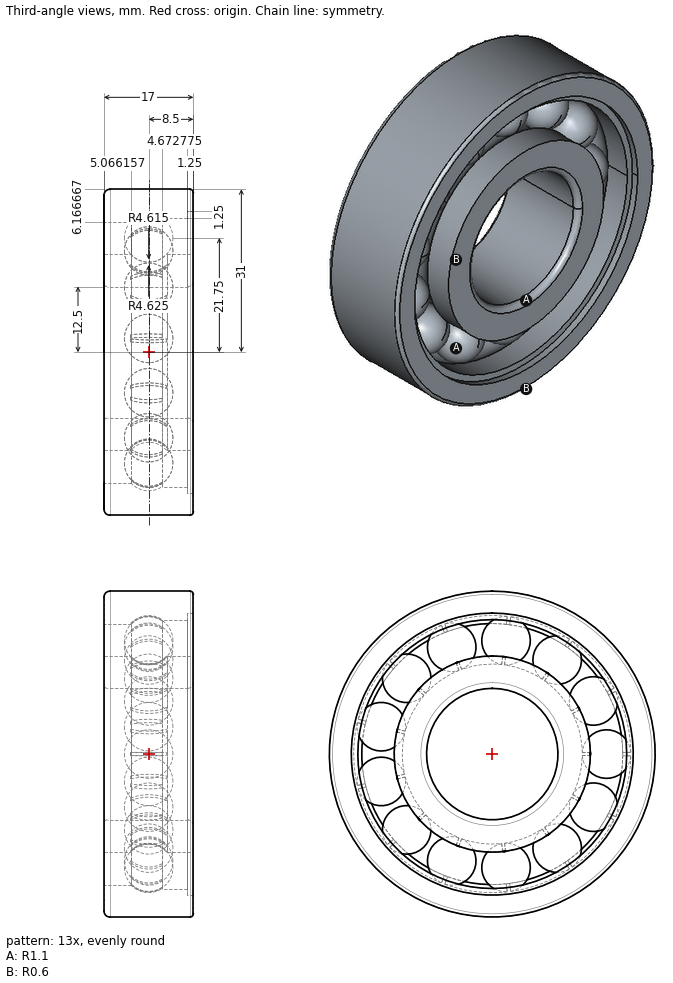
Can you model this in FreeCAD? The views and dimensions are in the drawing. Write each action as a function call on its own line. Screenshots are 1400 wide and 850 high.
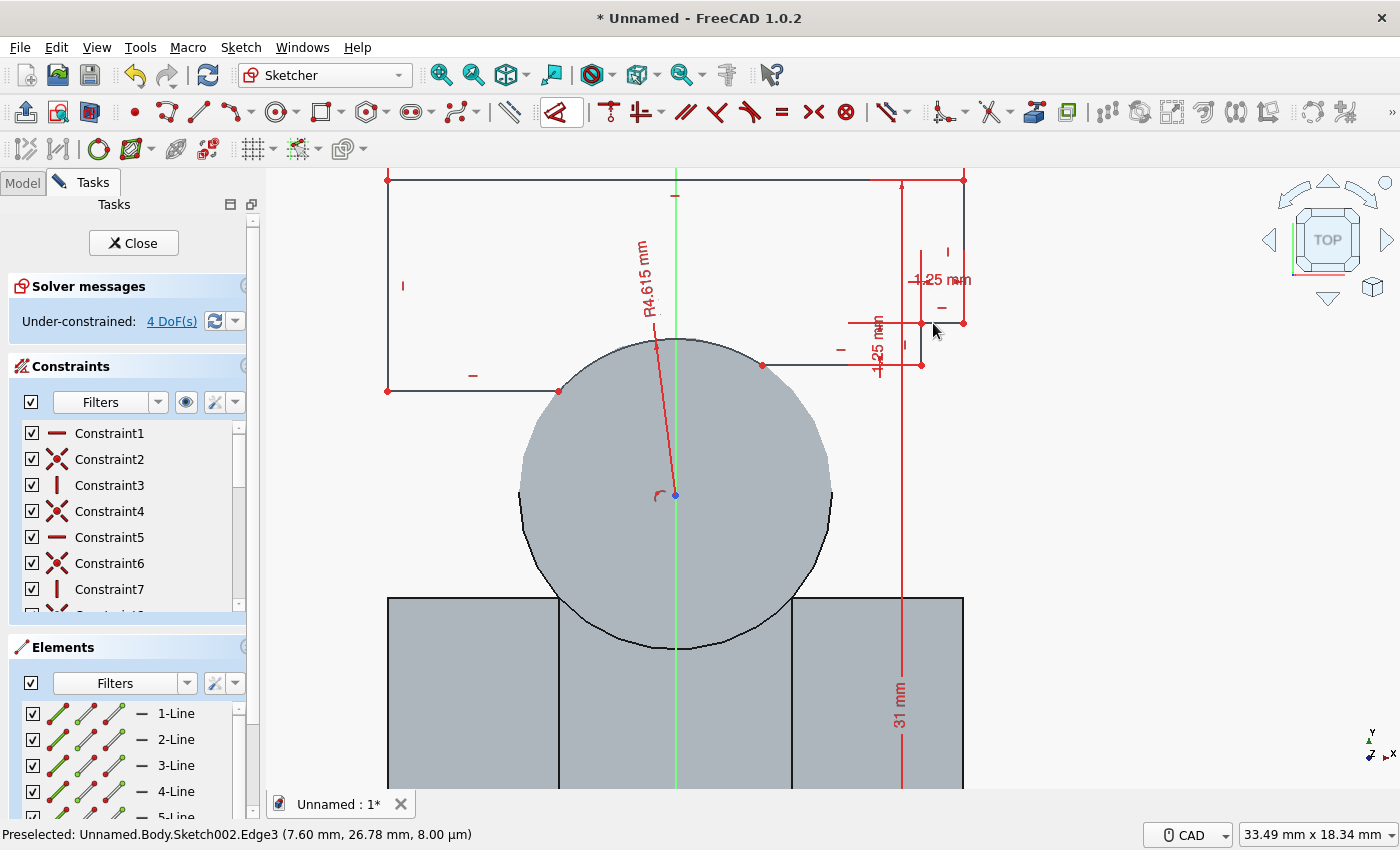
click(964, 323)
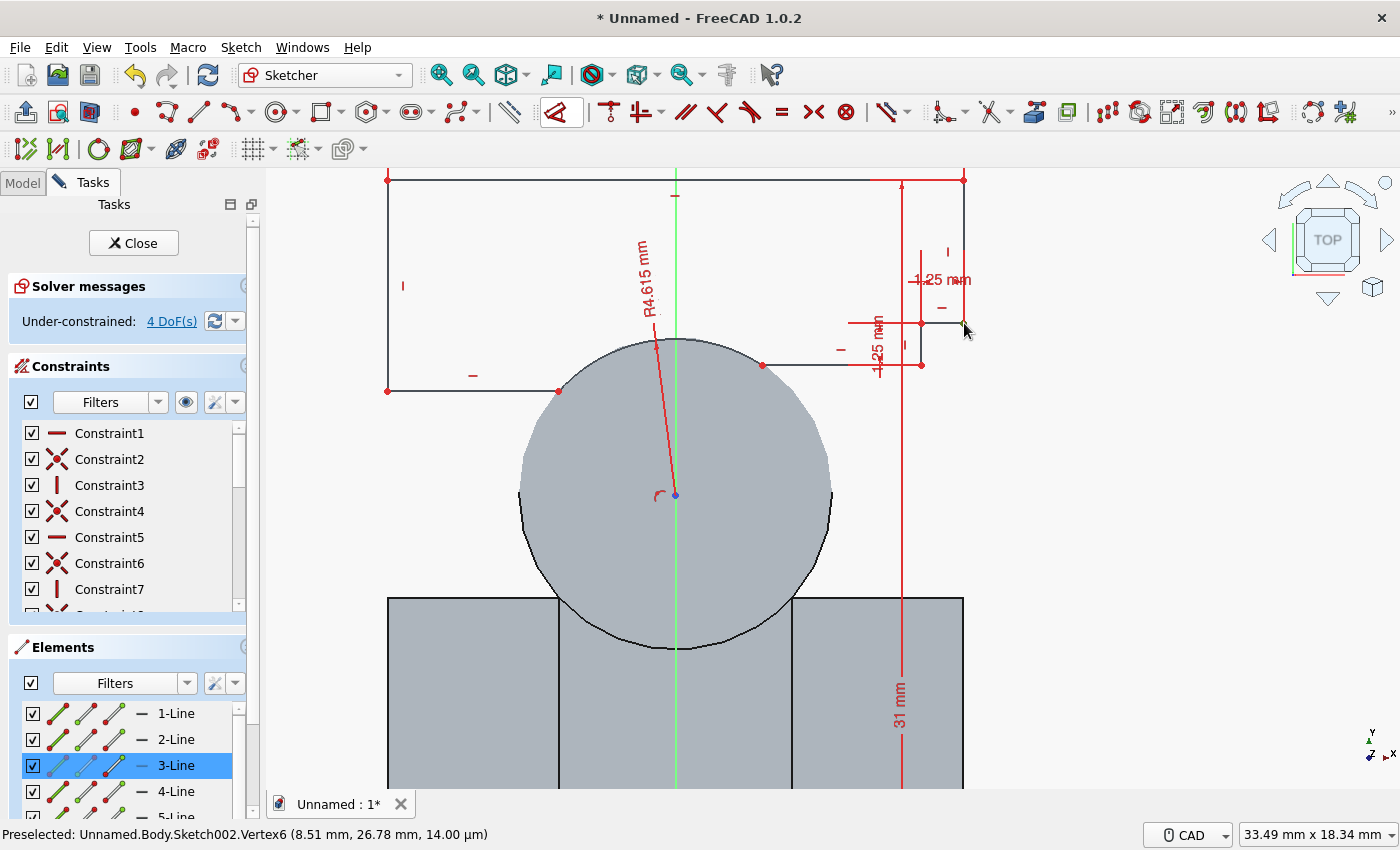
key(l)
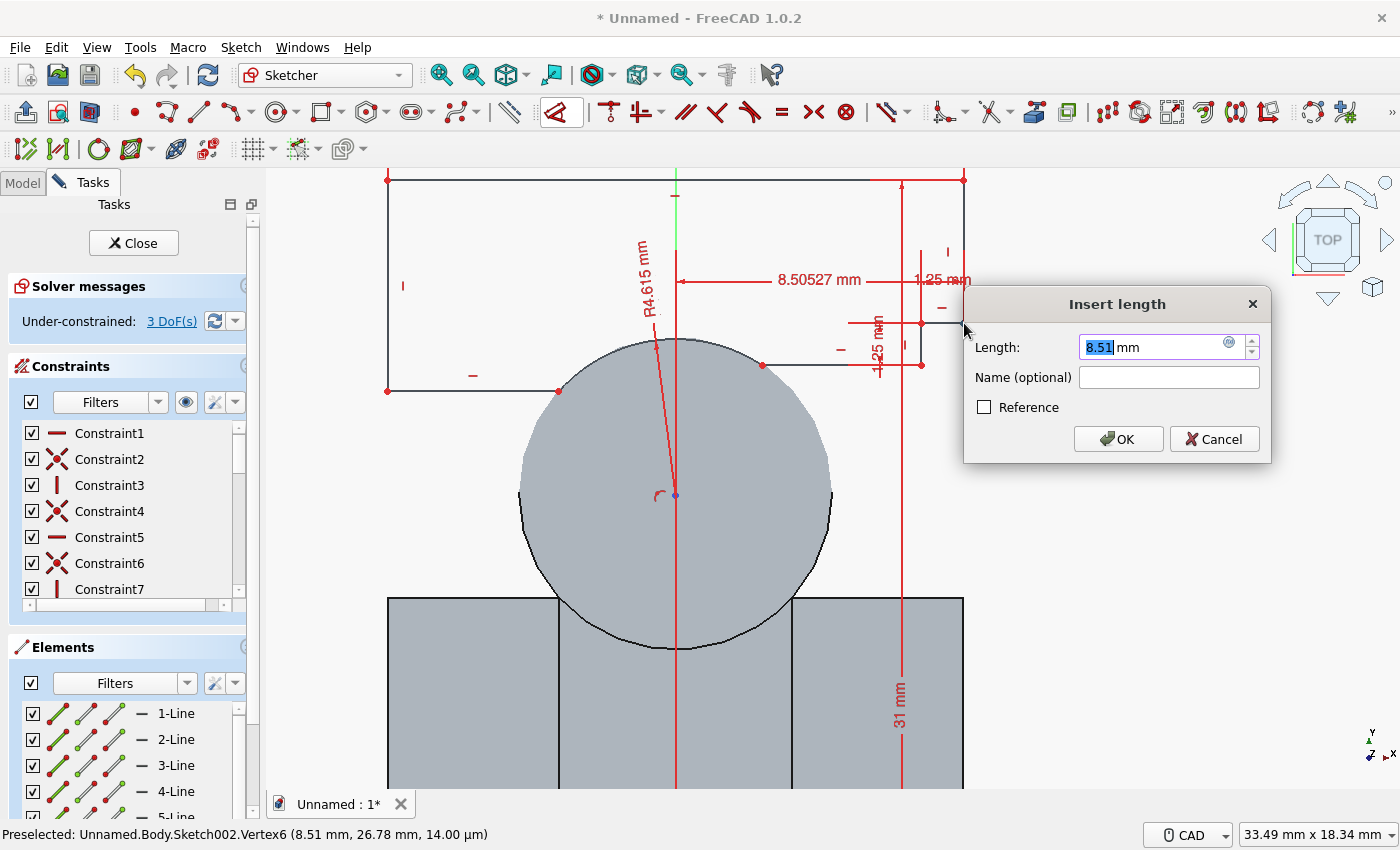
text(8.5)
key(Return)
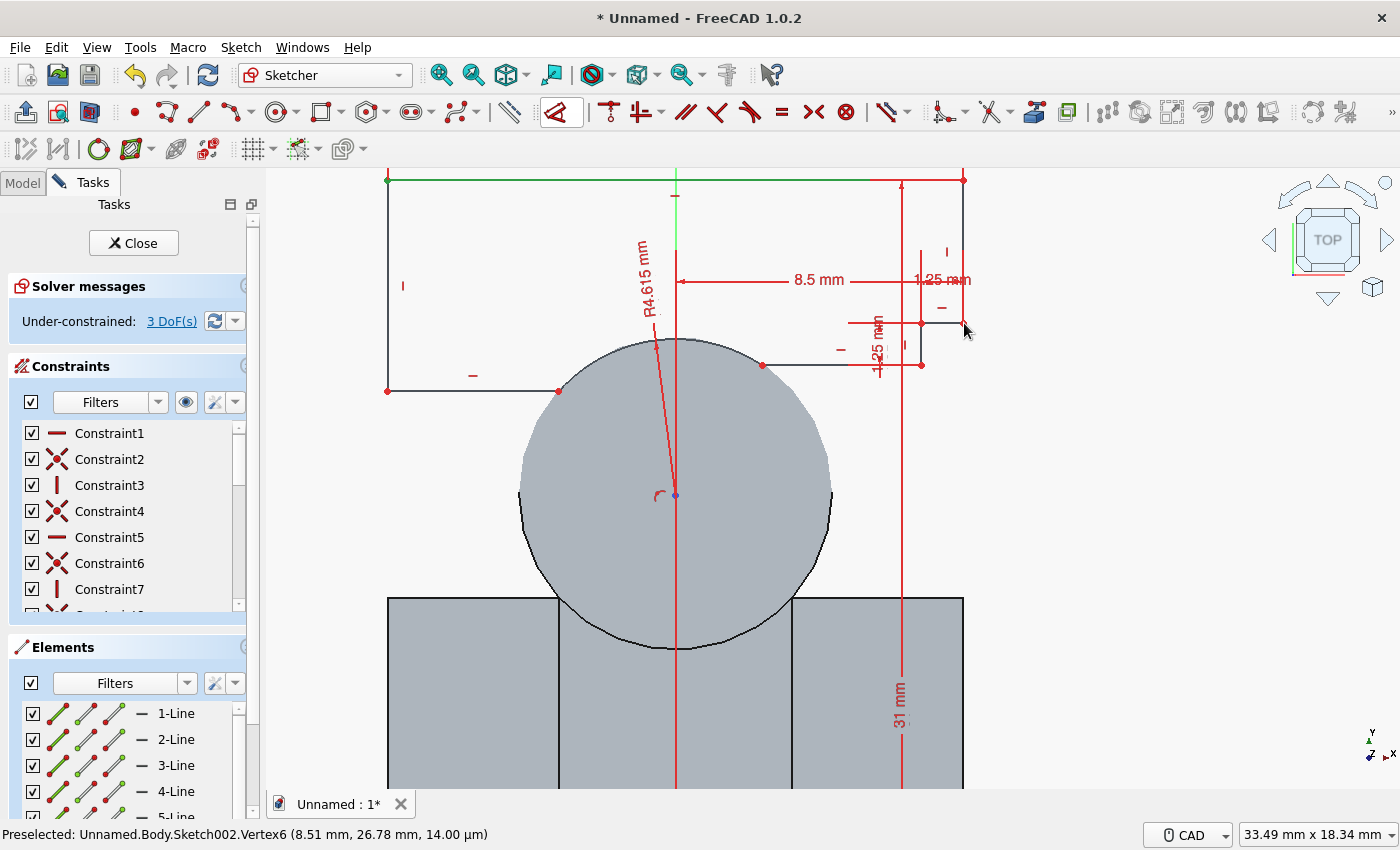
click(676, 495)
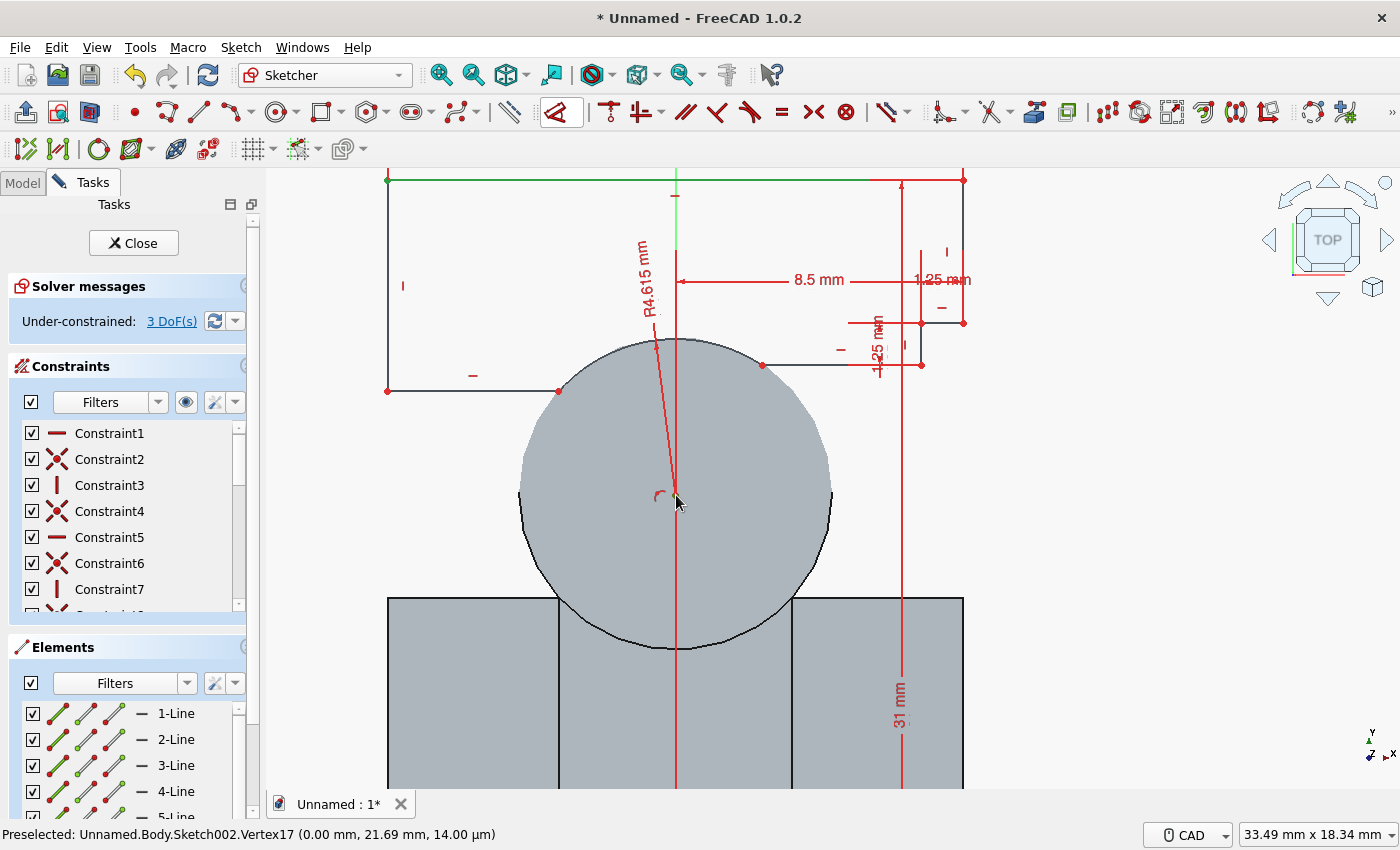
key(i)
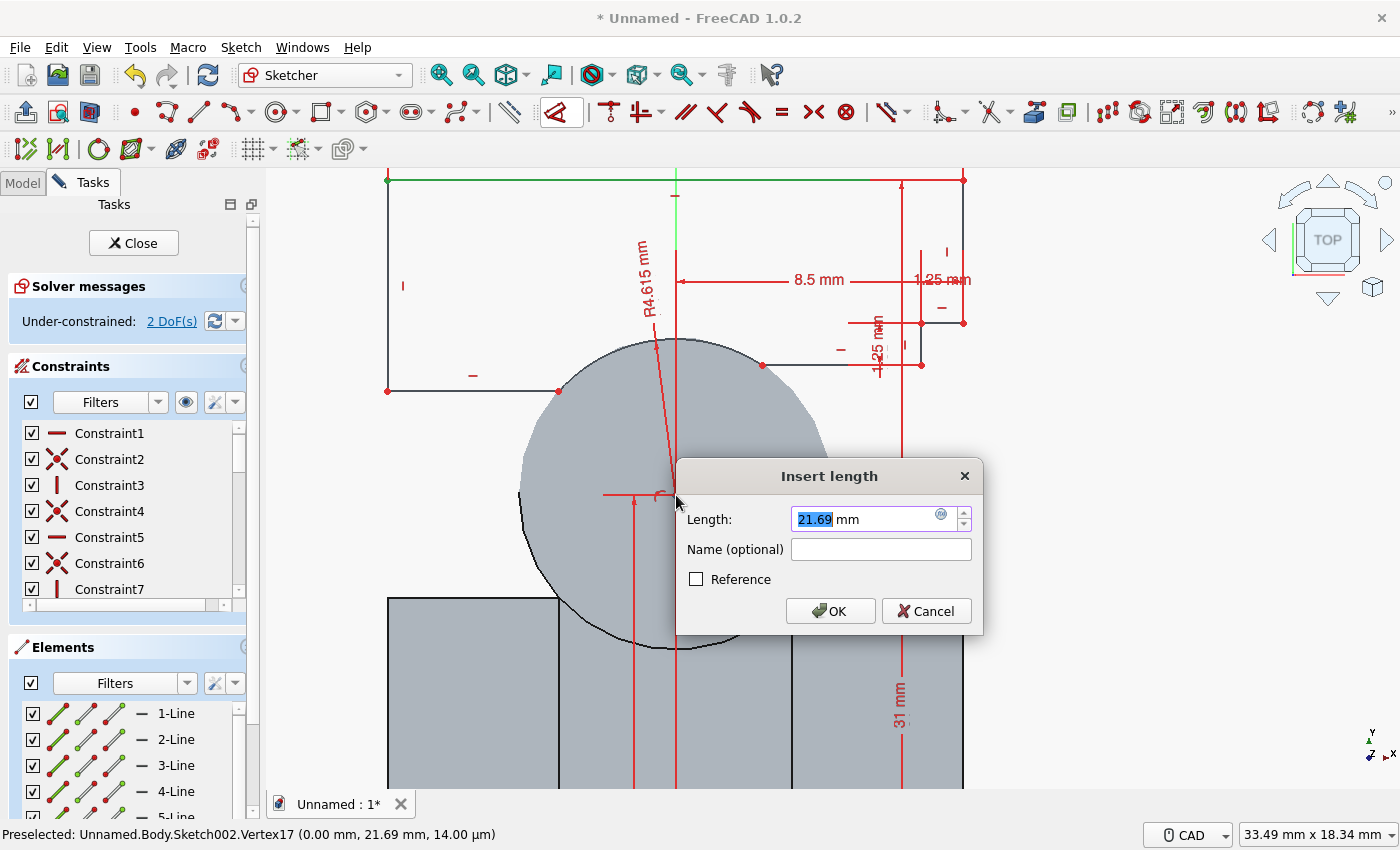
text(21.75)
key(Return)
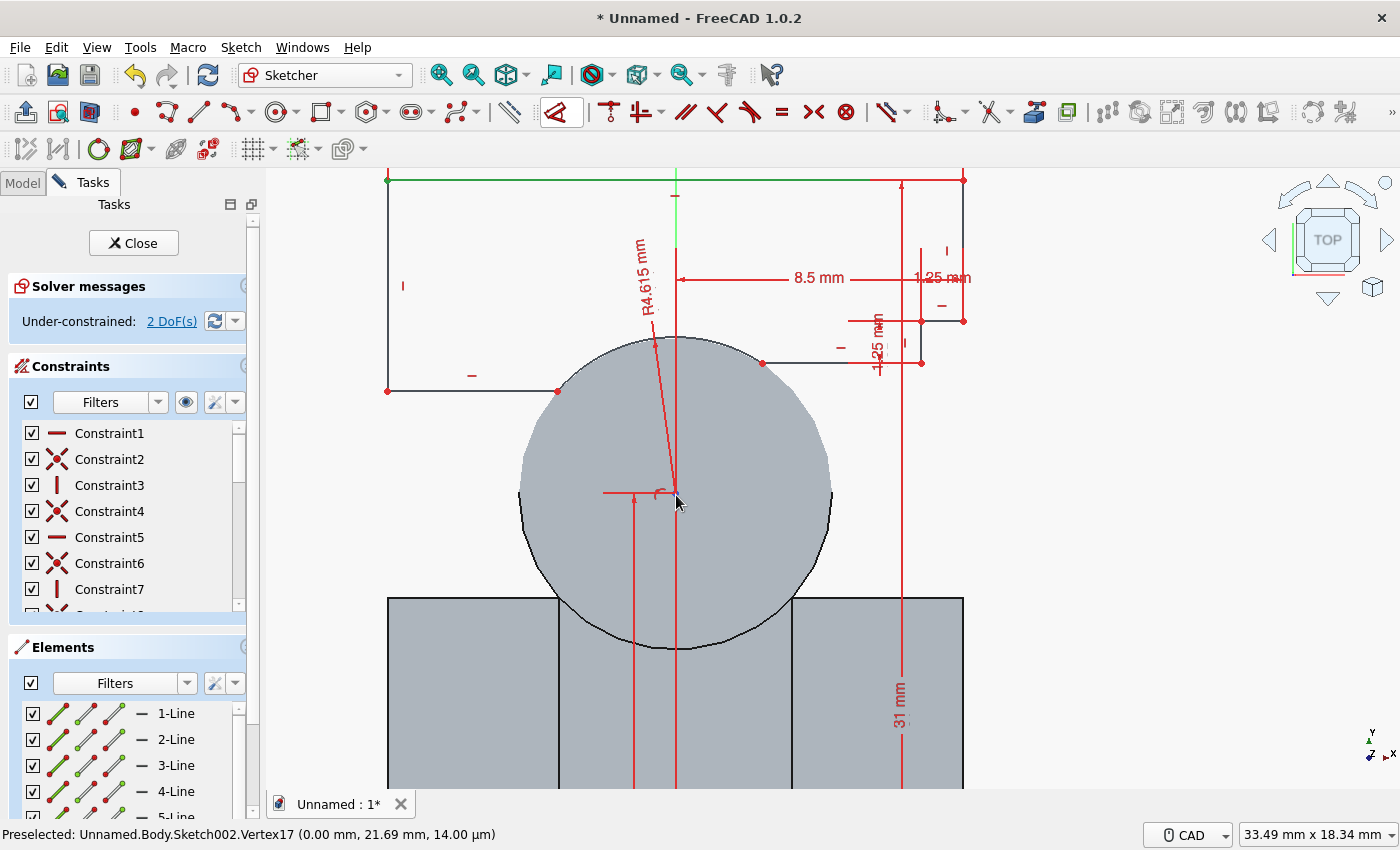
click(810, 363)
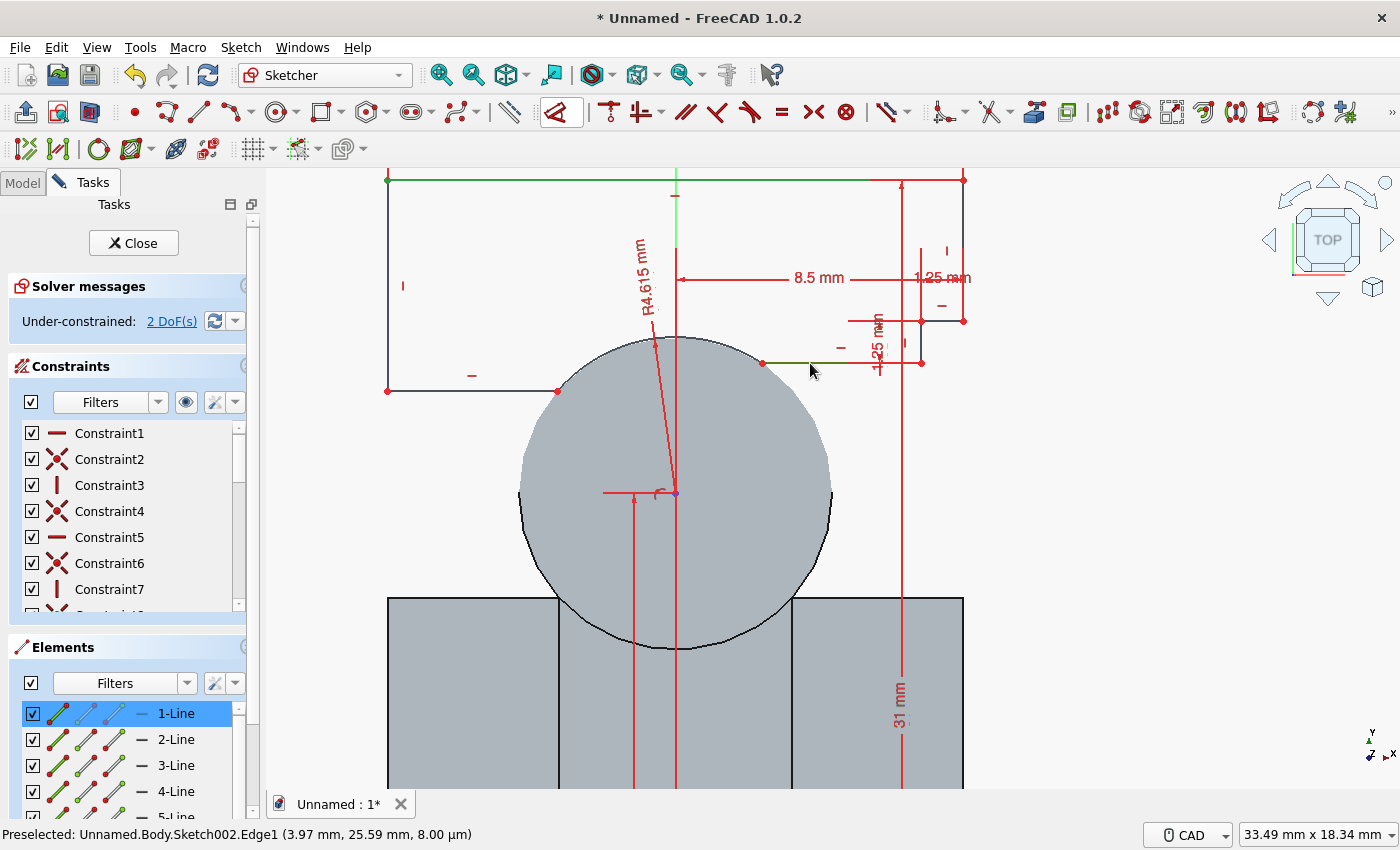
key(l)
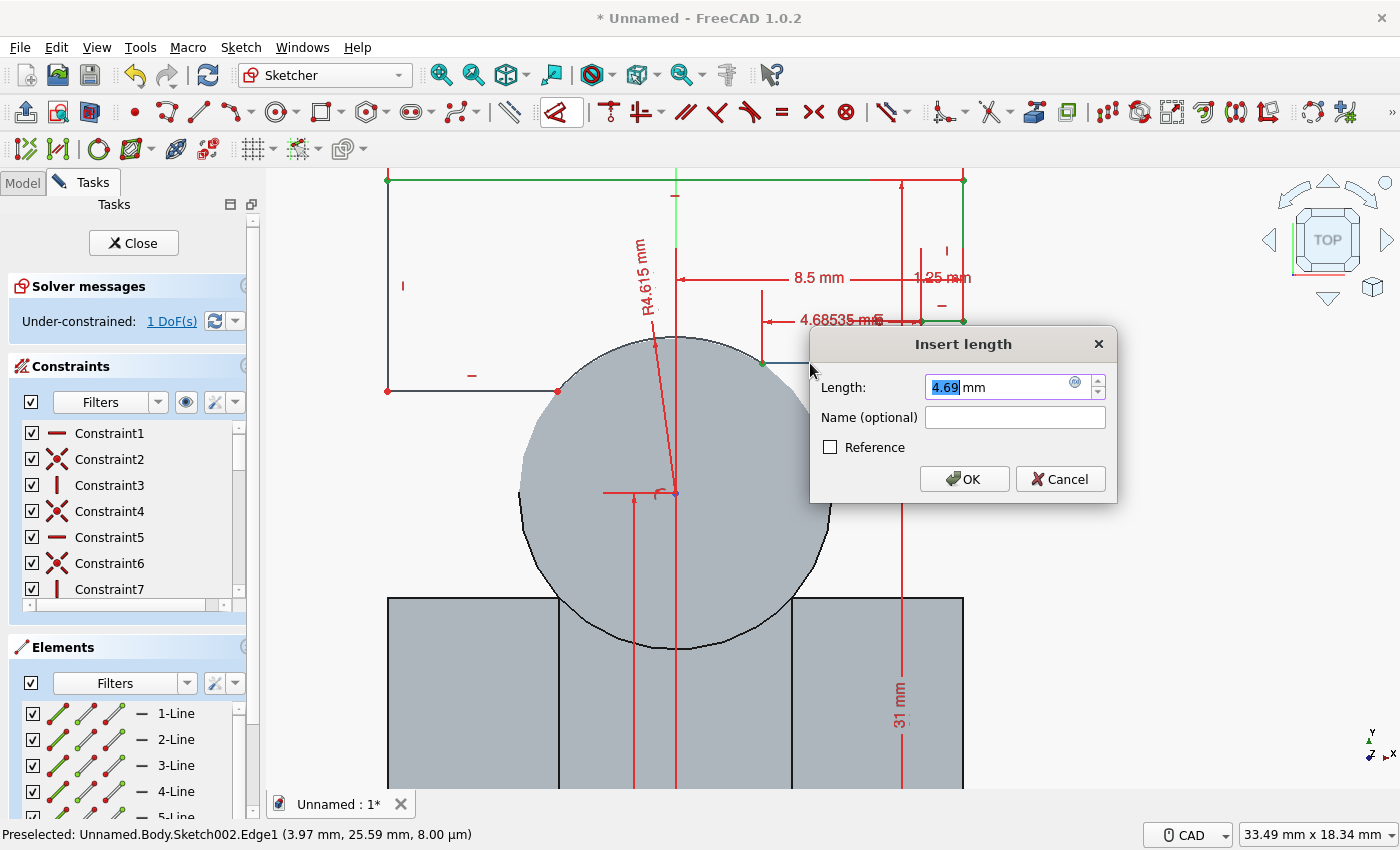
text(4.672775)
key(Return)